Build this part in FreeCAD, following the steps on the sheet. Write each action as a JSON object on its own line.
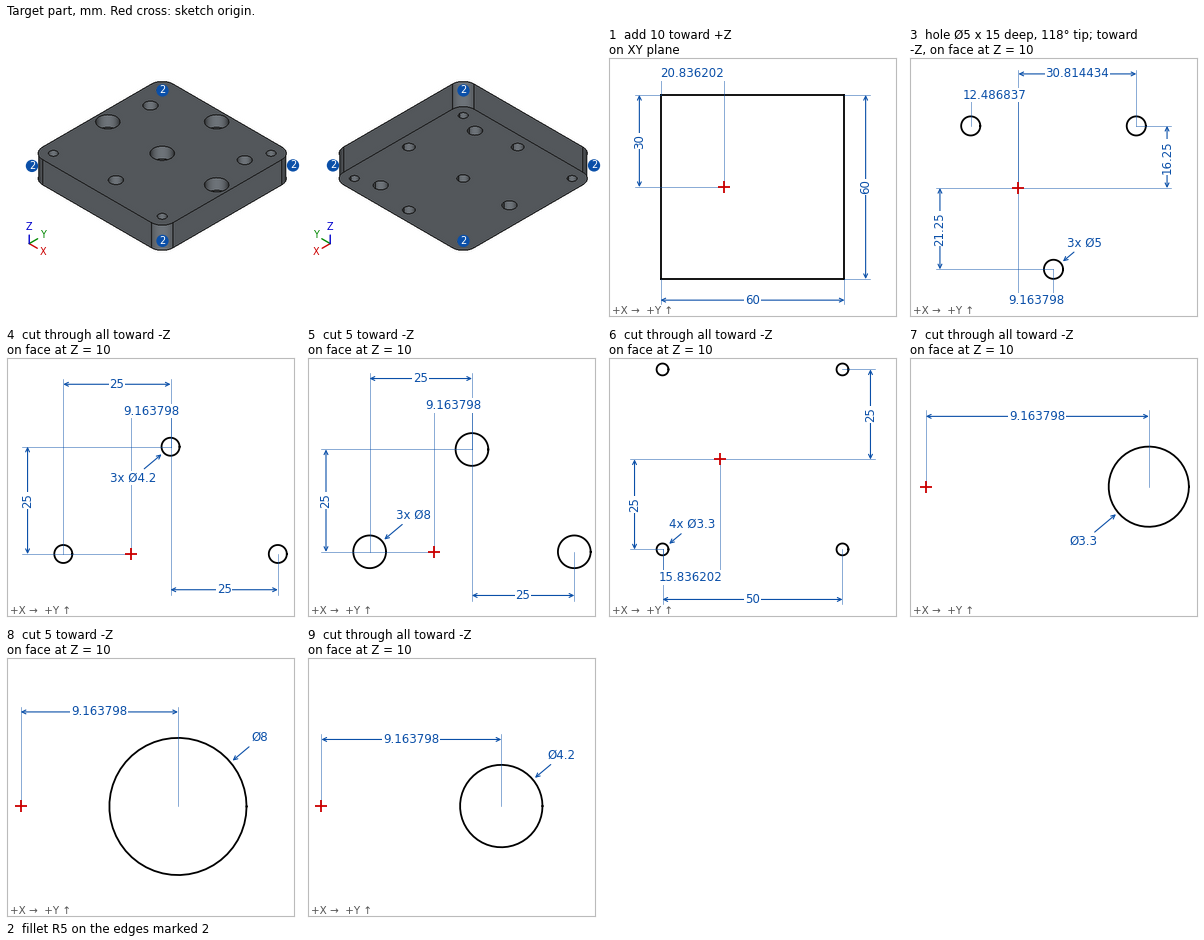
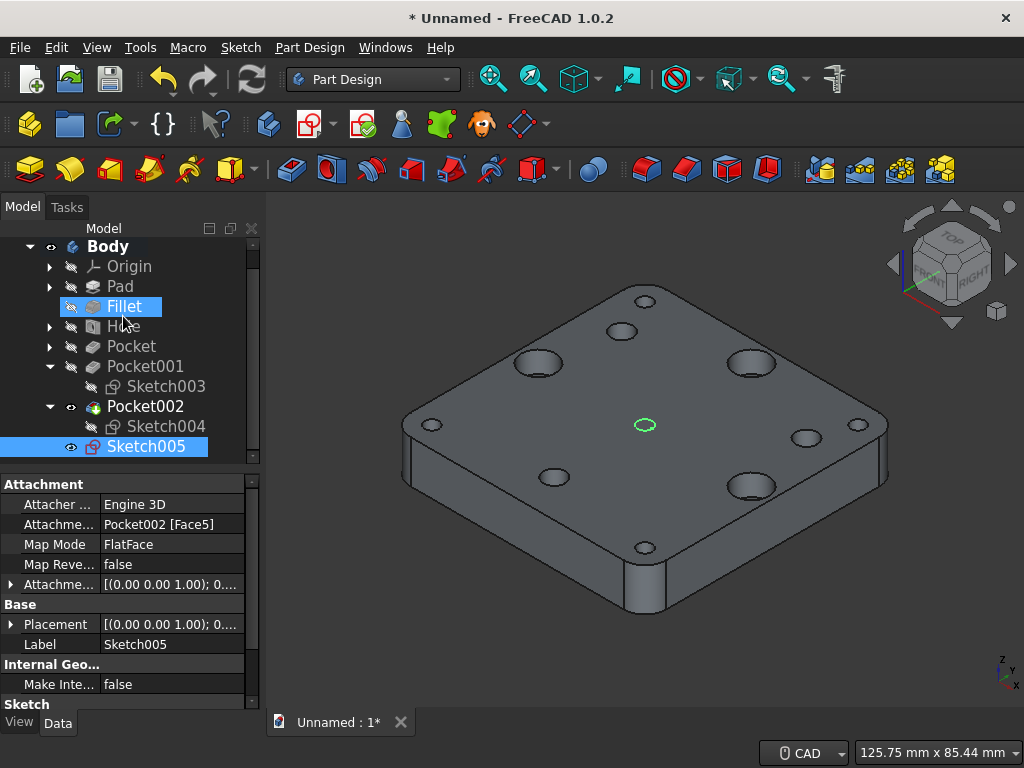
{"action": "left_click", "coordinate": [292, 170]}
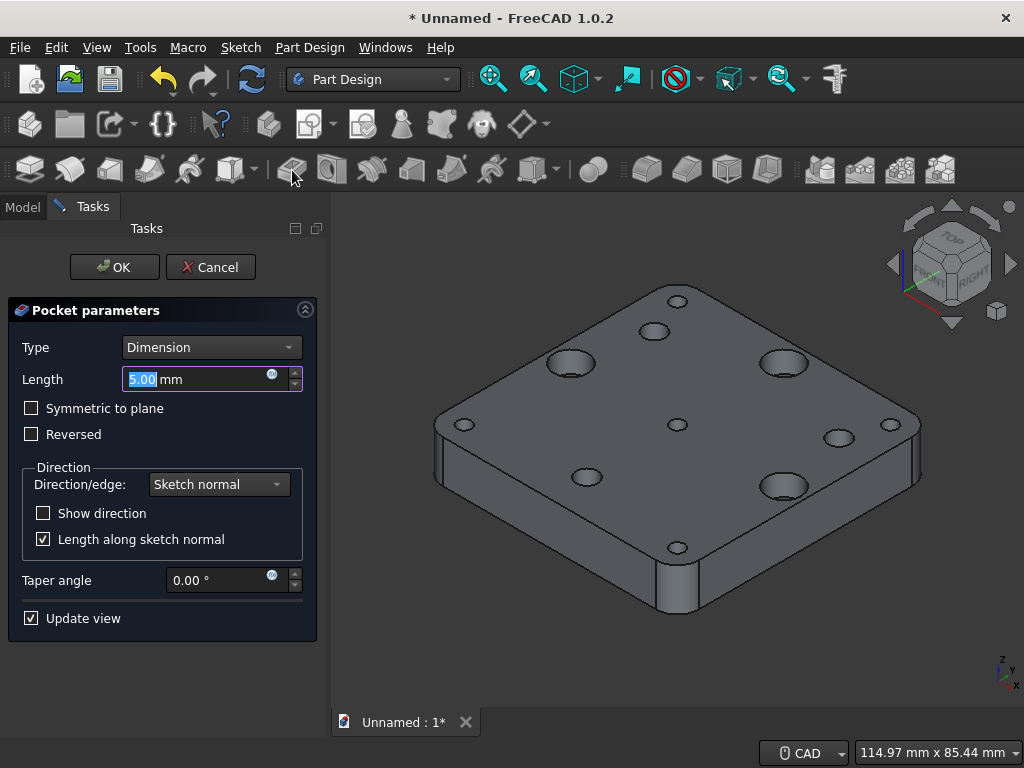
{"action": "left_click", "coordinate": [212, 348]}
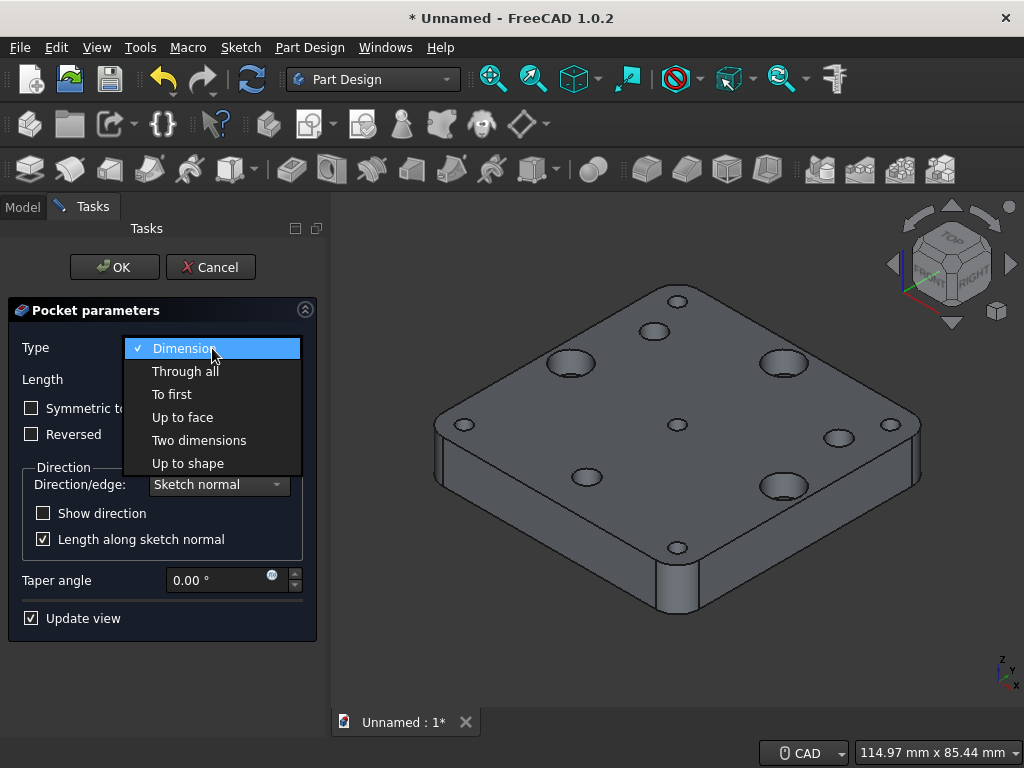
{"action": "left_click", "coordinate": [212, 372]}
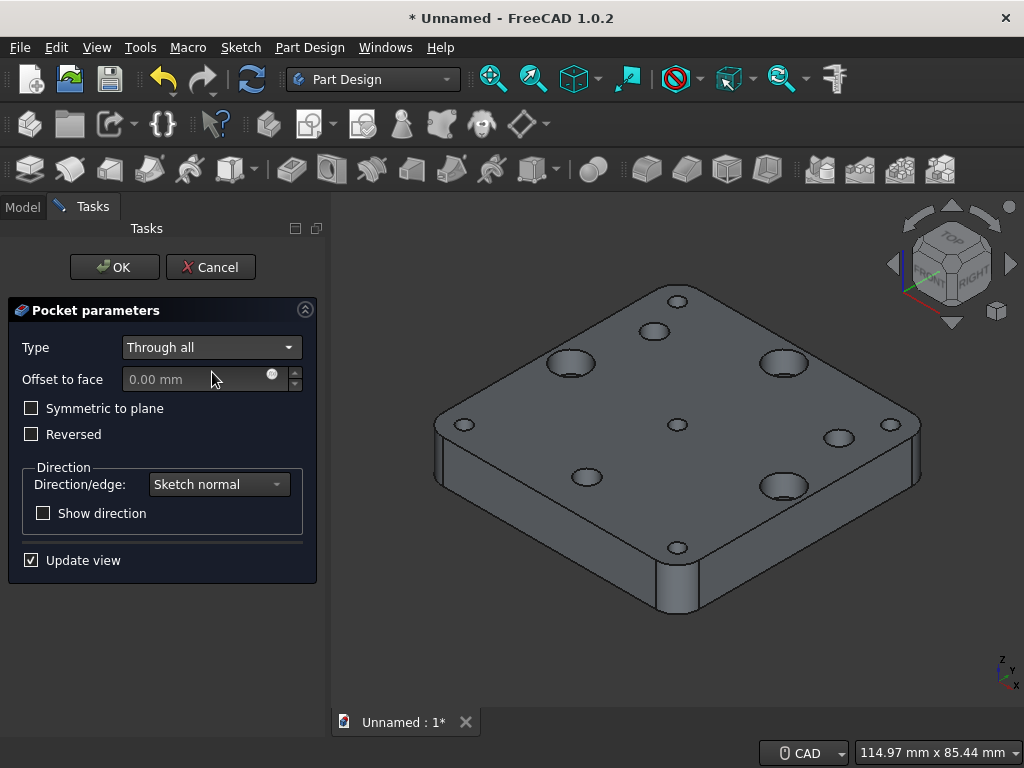
{"action": "left_click", "coordinate": [115, 267]}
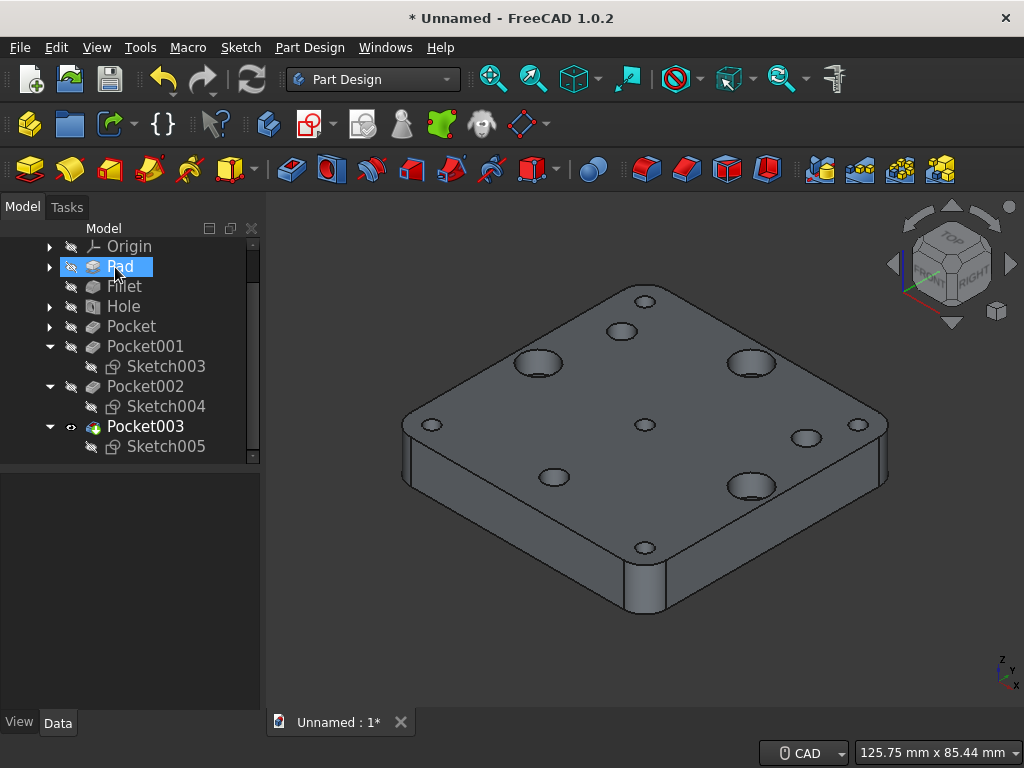
{"action": "left_click", "coordinate": [572, 424]}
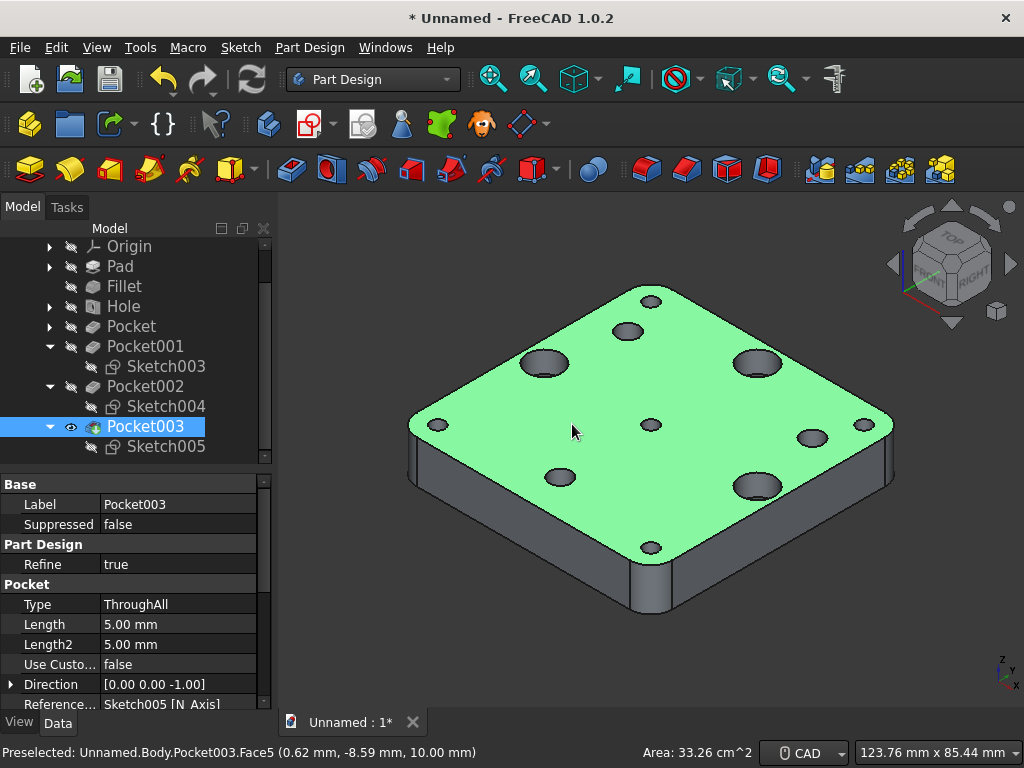
{"action": "left_click", "coordinate": [310, 124]}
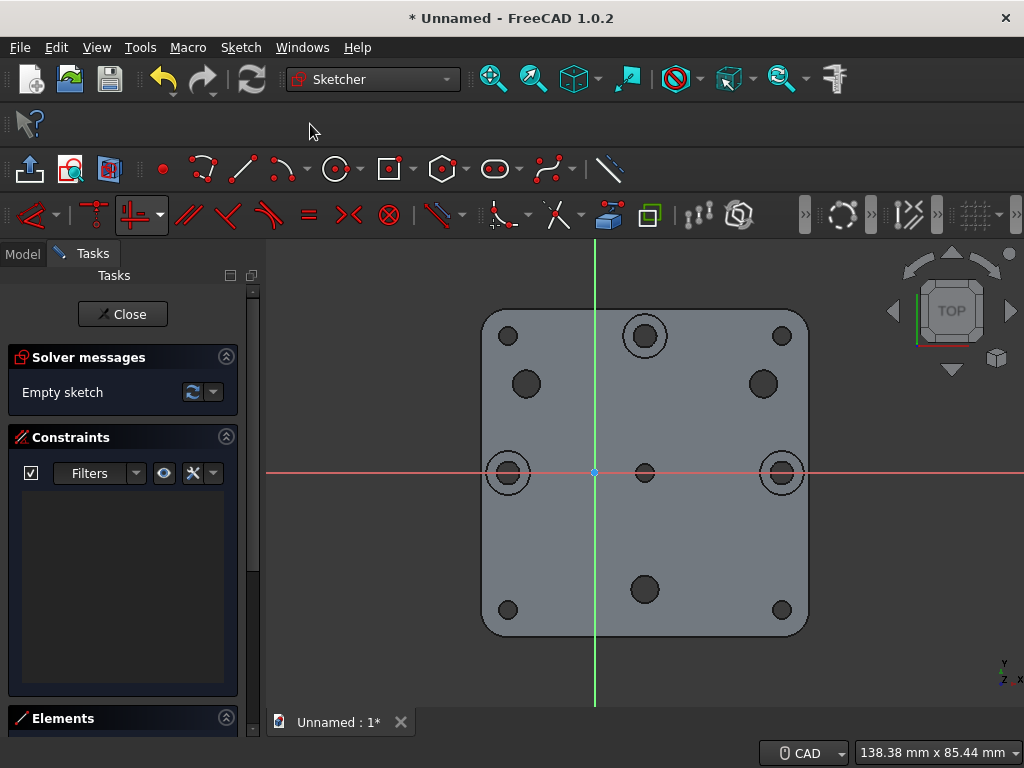
{"action": "scroll", "coordinate": [642, 473], "scroll_direction": "up", "scroll_amount": 9}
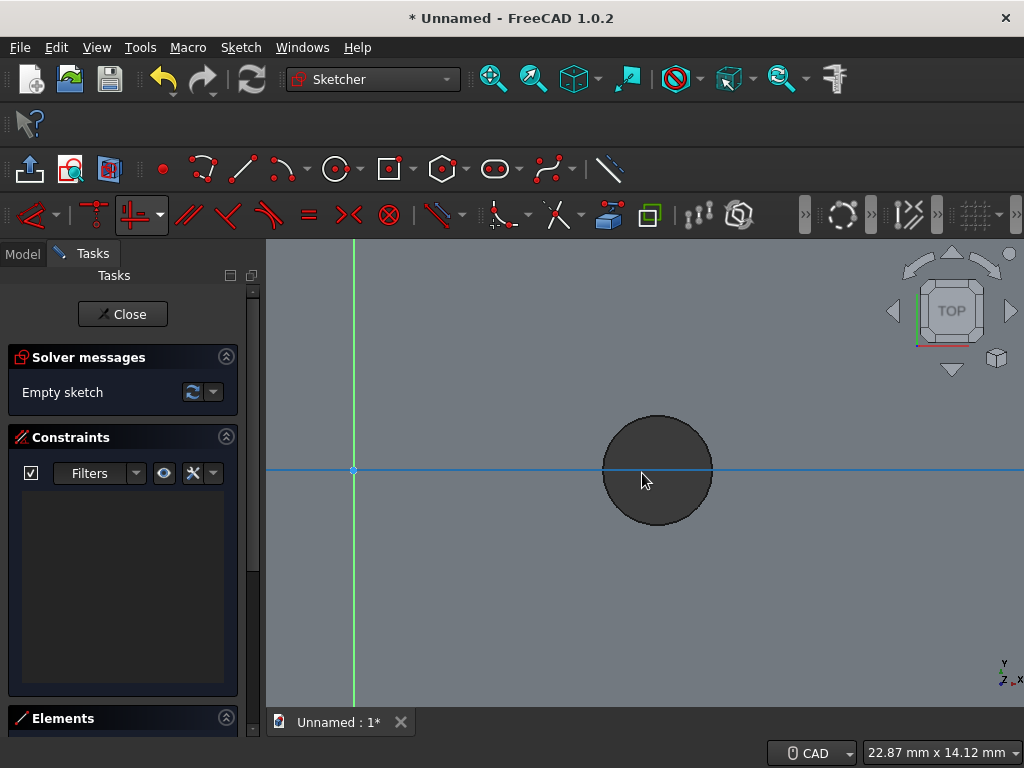
{"action": "left_click", "coordinate": [336, 170]}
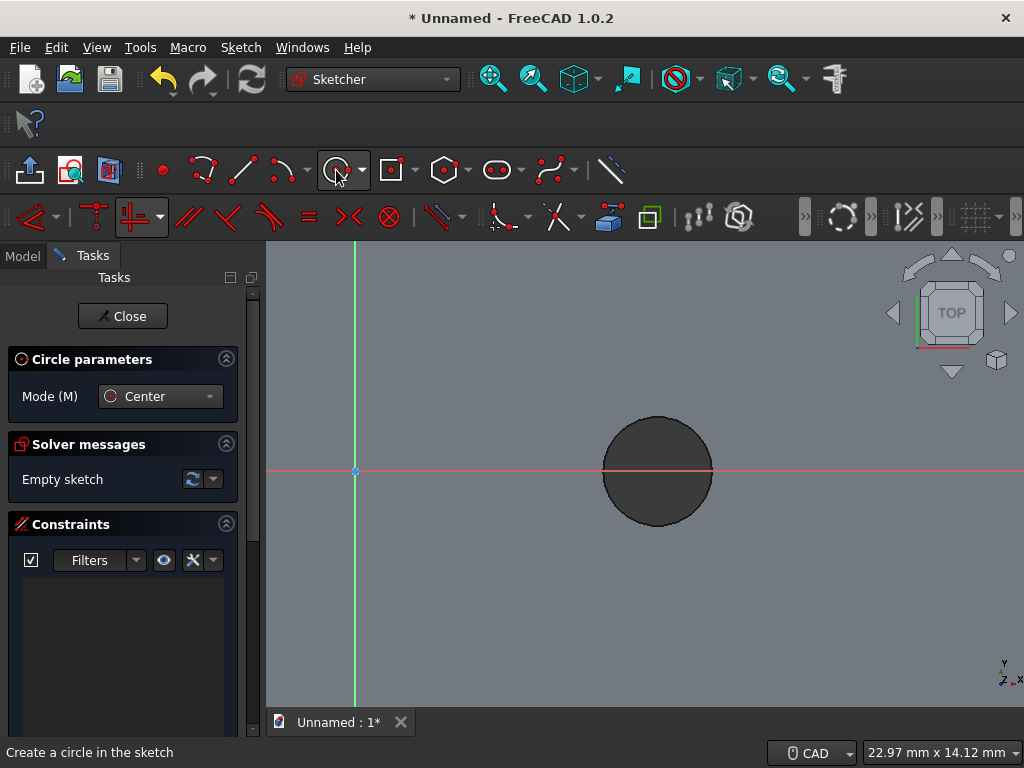
{"action": "left_click", "coordinate": [658, 471]}
{"action": "mouse_move", "coordinate": [751, 378]}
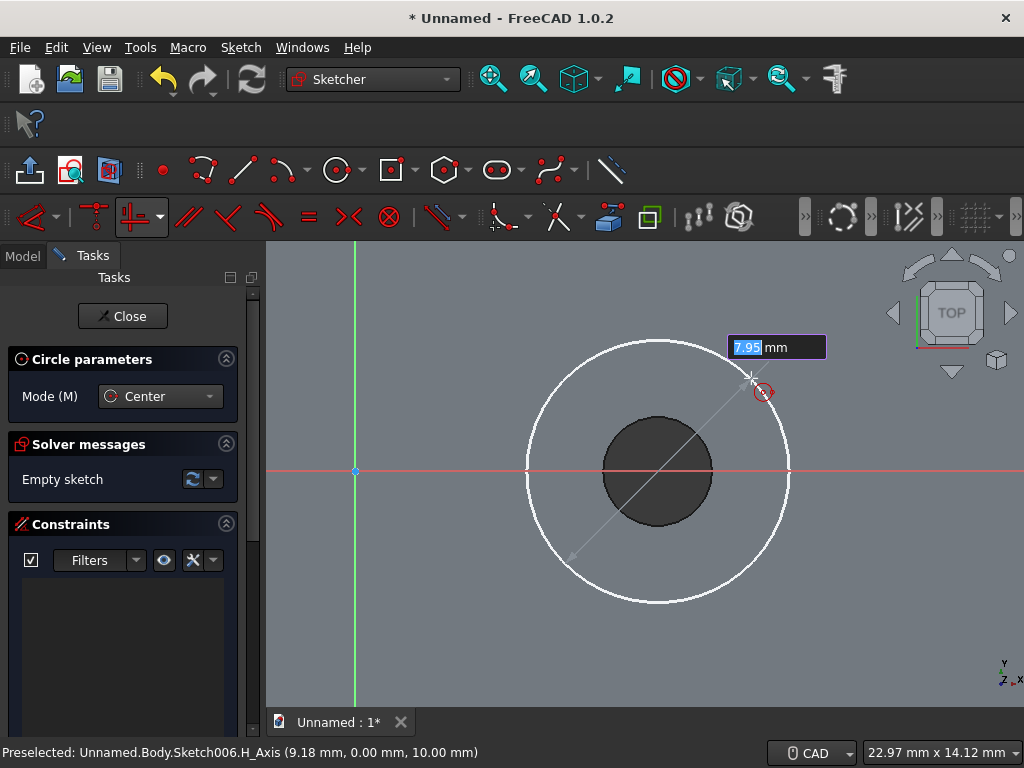
{"action": "type", "text": "8"}
{"action": "key", "text": "Return"}
{"action": "key", "text": "Escape"}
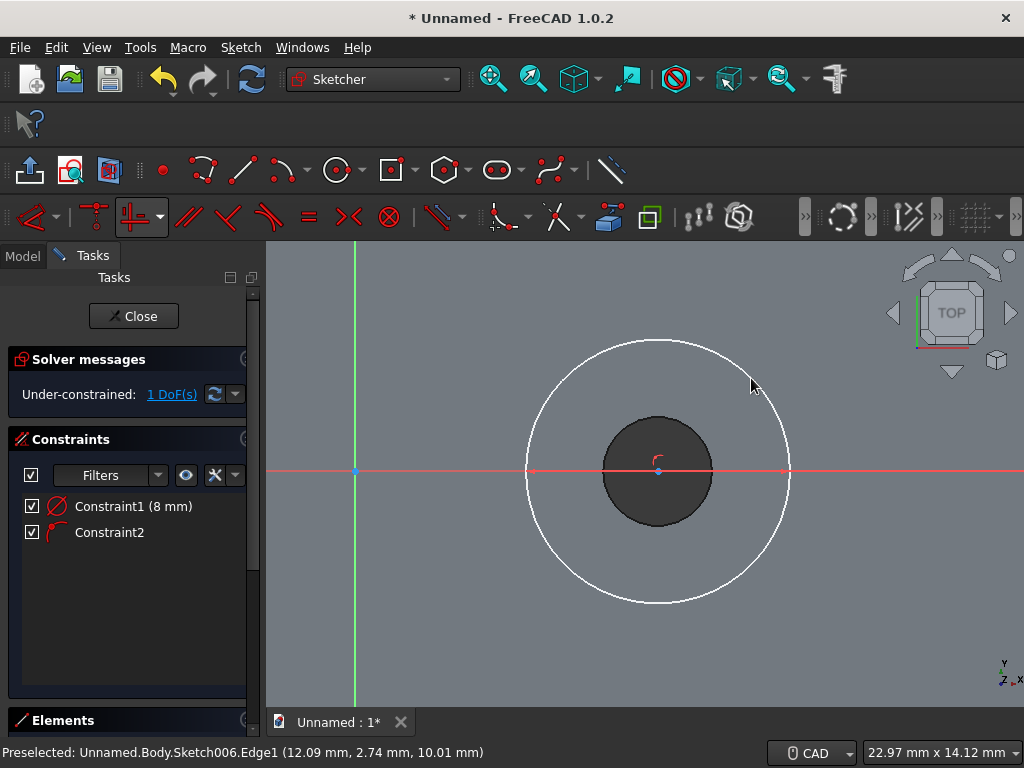
{"action": "left_click", "coordinate": [32, 218]}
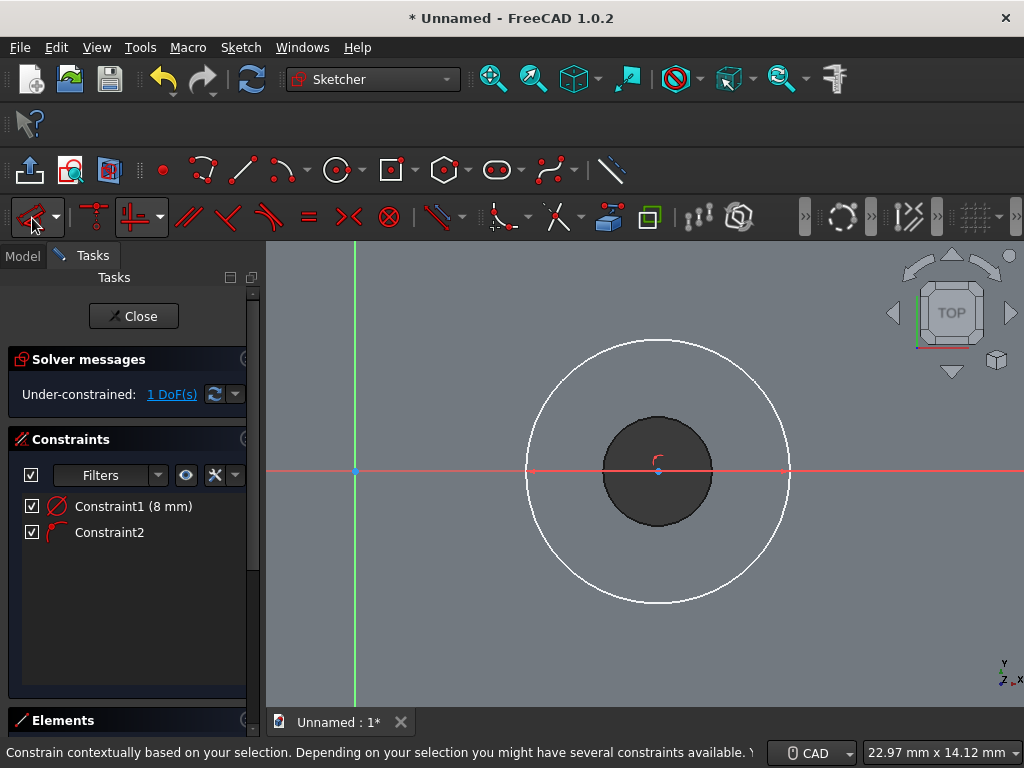
{"action": "left_click", "coordinate": [658, 471]}
{"action": "left_click", "coordinate": [507, 505]}